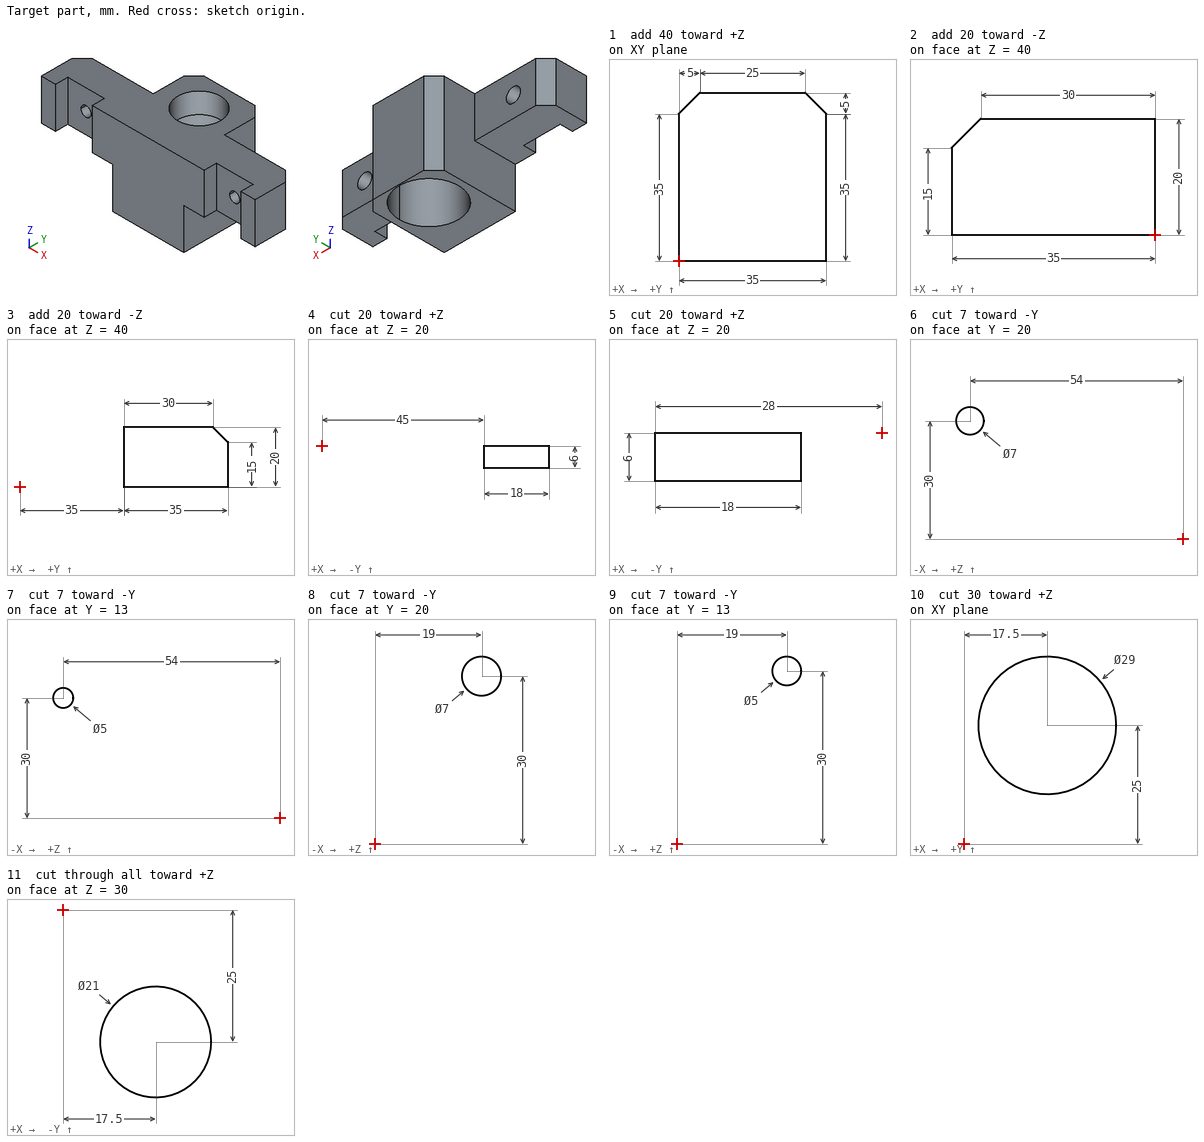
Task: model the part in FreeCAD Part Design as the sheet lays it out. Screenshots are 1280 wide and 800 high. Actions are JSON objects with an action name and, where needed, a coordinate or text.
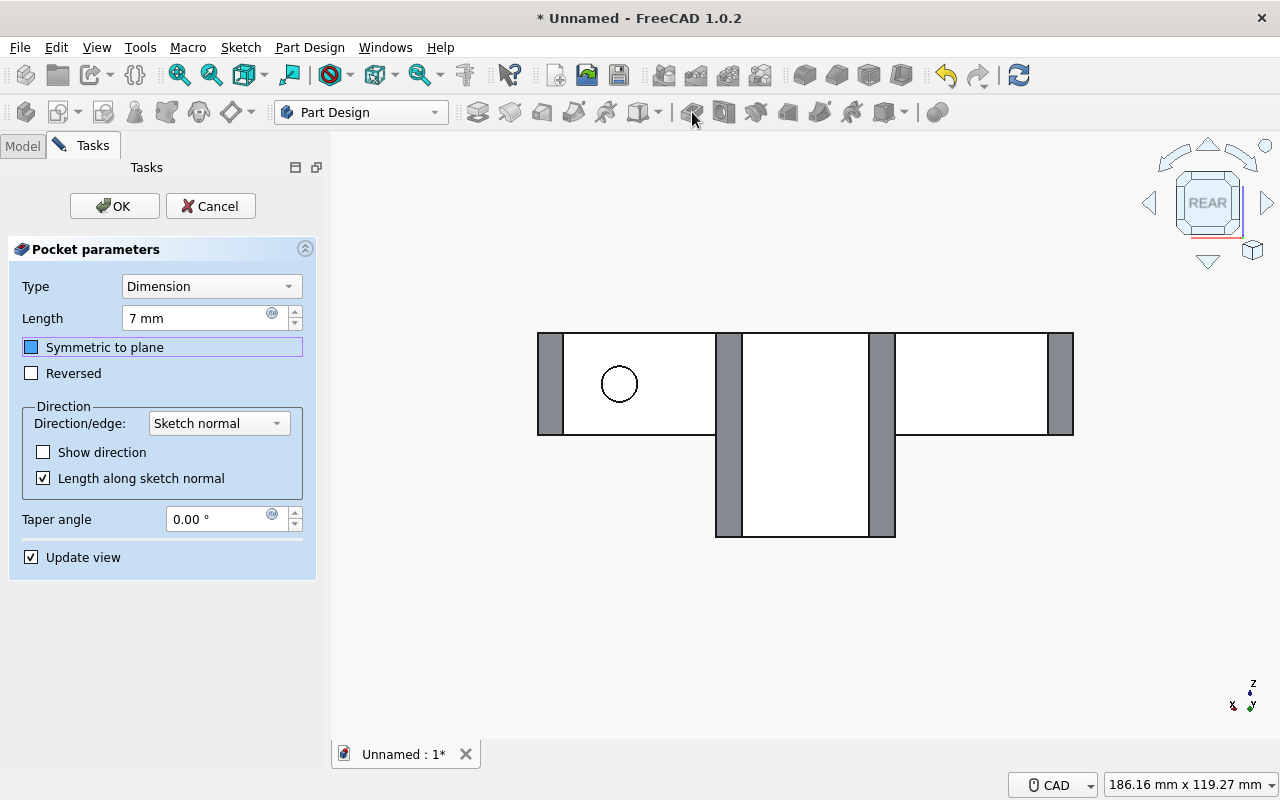
{"action": "left_click", "coordinate": [115, 206]}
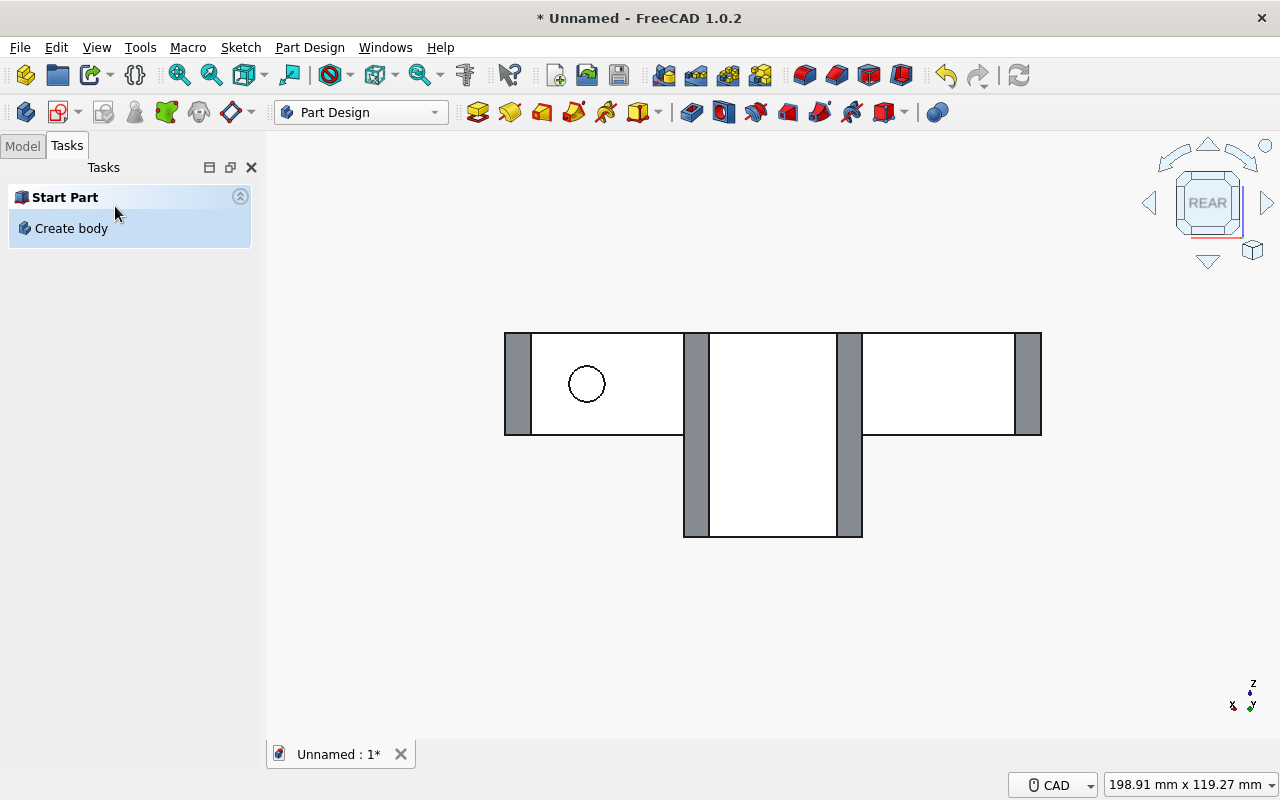
{"action": "left_click", "coordinate": [587, 383]}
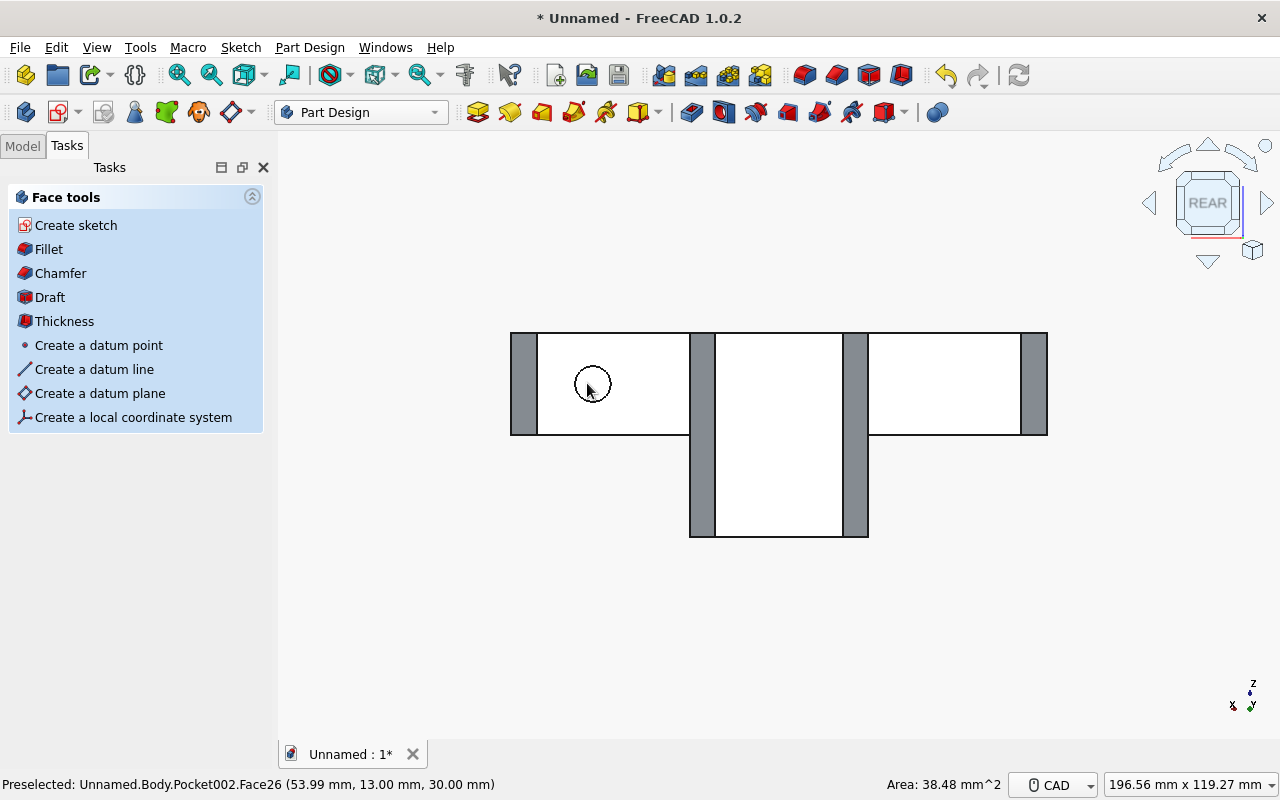
{"action": "left_click", "coordinate": [58, 112]}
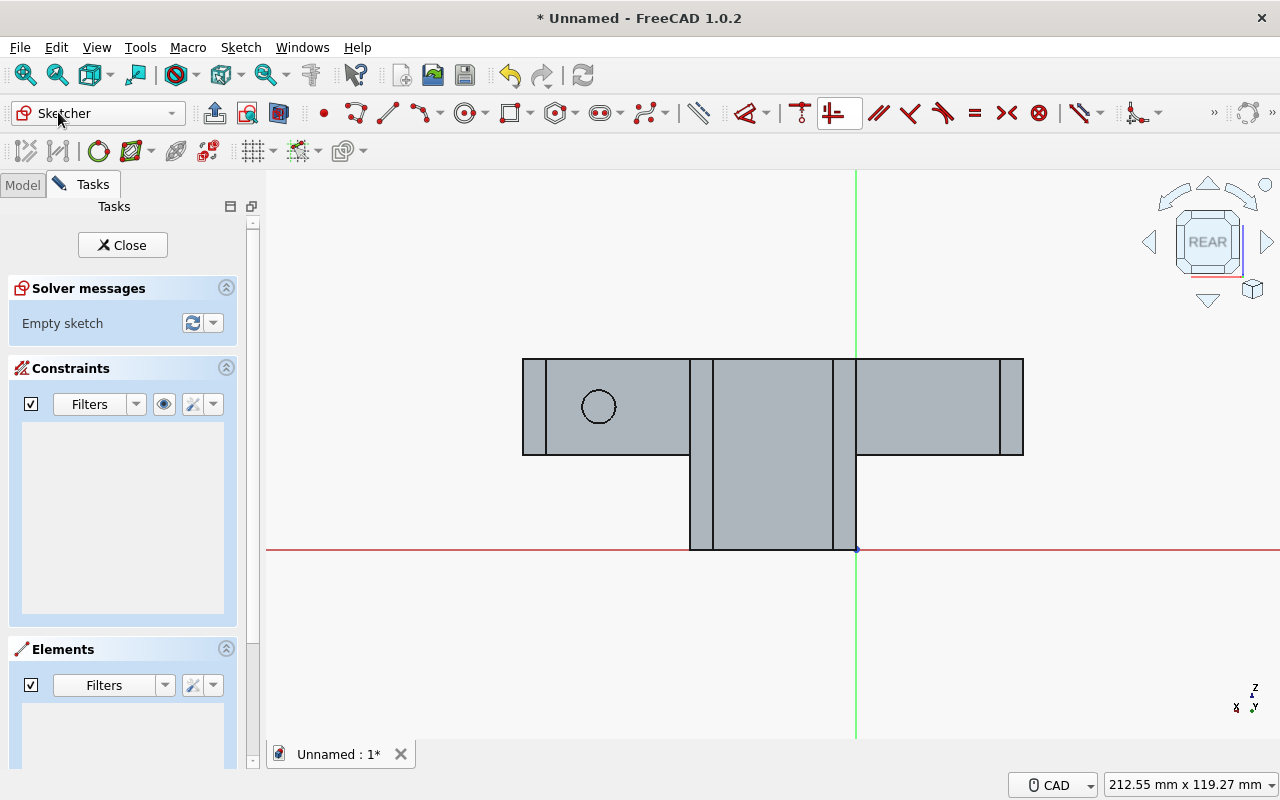
{"action": "scroll", "coordinate": [592, 404], "scroll_direction": "up", "scroll_amount": 14}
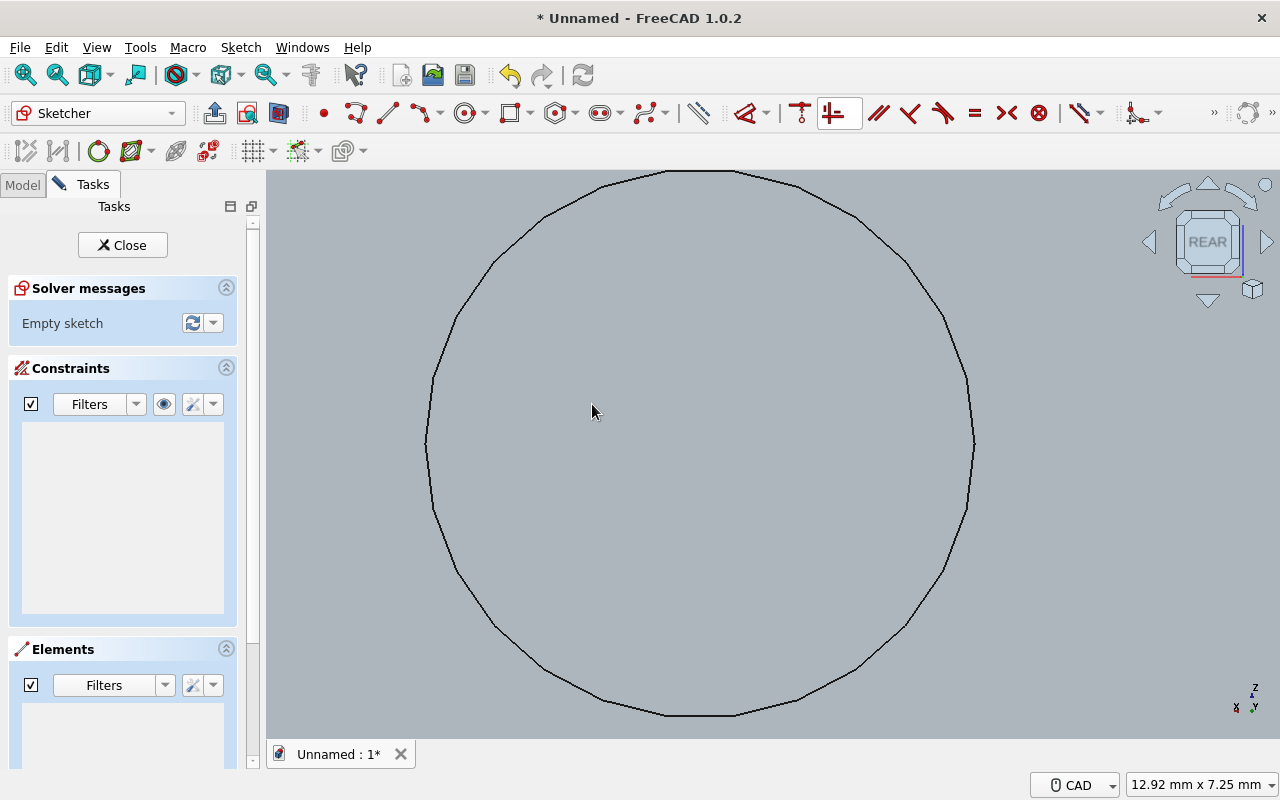
{"action": "left_click", "coordinate": [466, 114]}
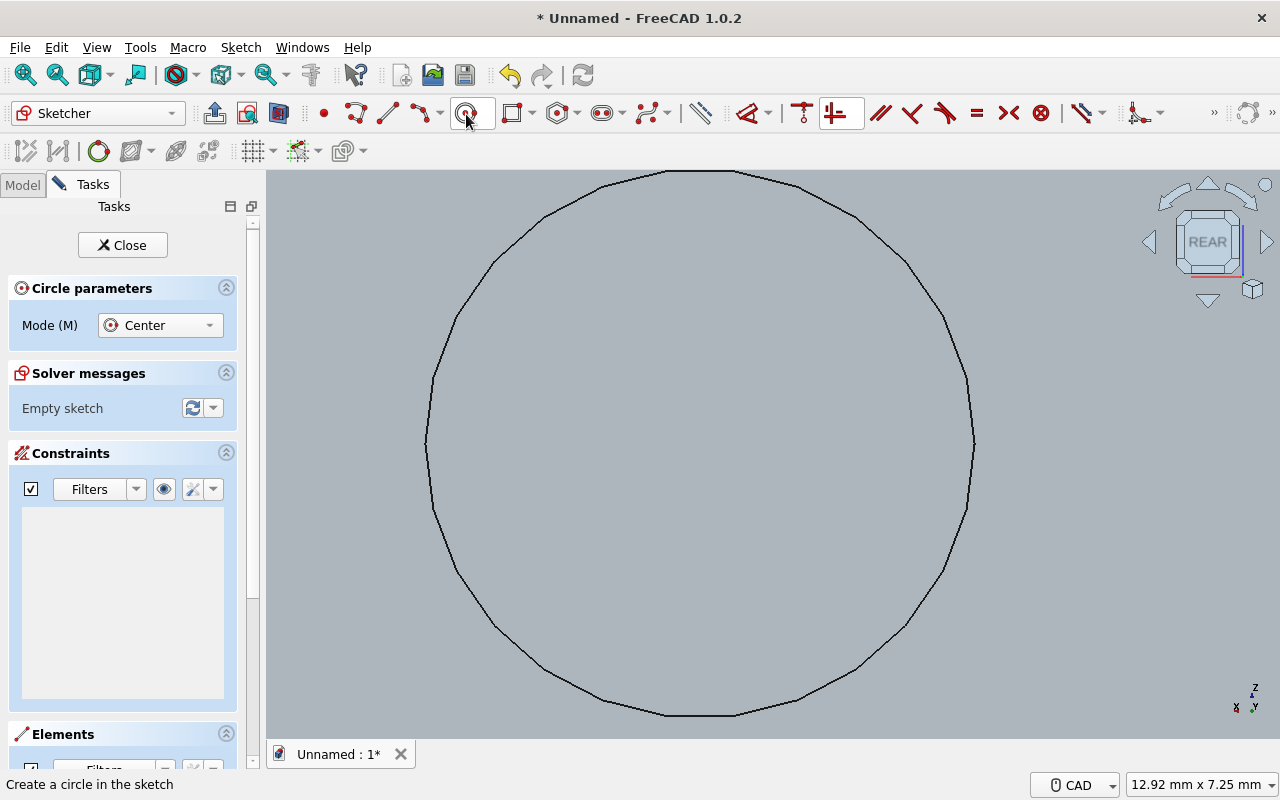
{"action": "left_click", "coordinate": [700, 444]}
{"action": "left_click", "coordinate": [839, 305]}
{"action": "key", "text": "Escape"}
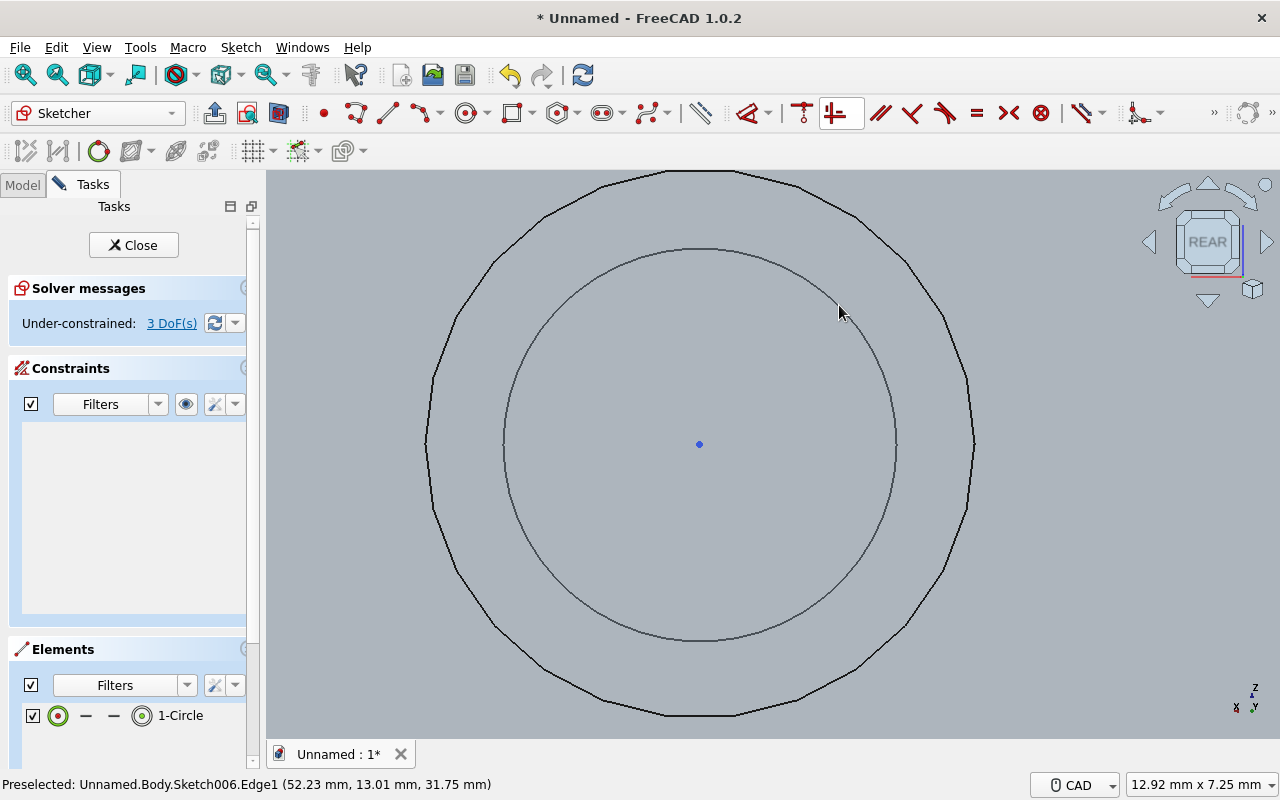
{"action": "left_click", "coordinate": [748, 114]}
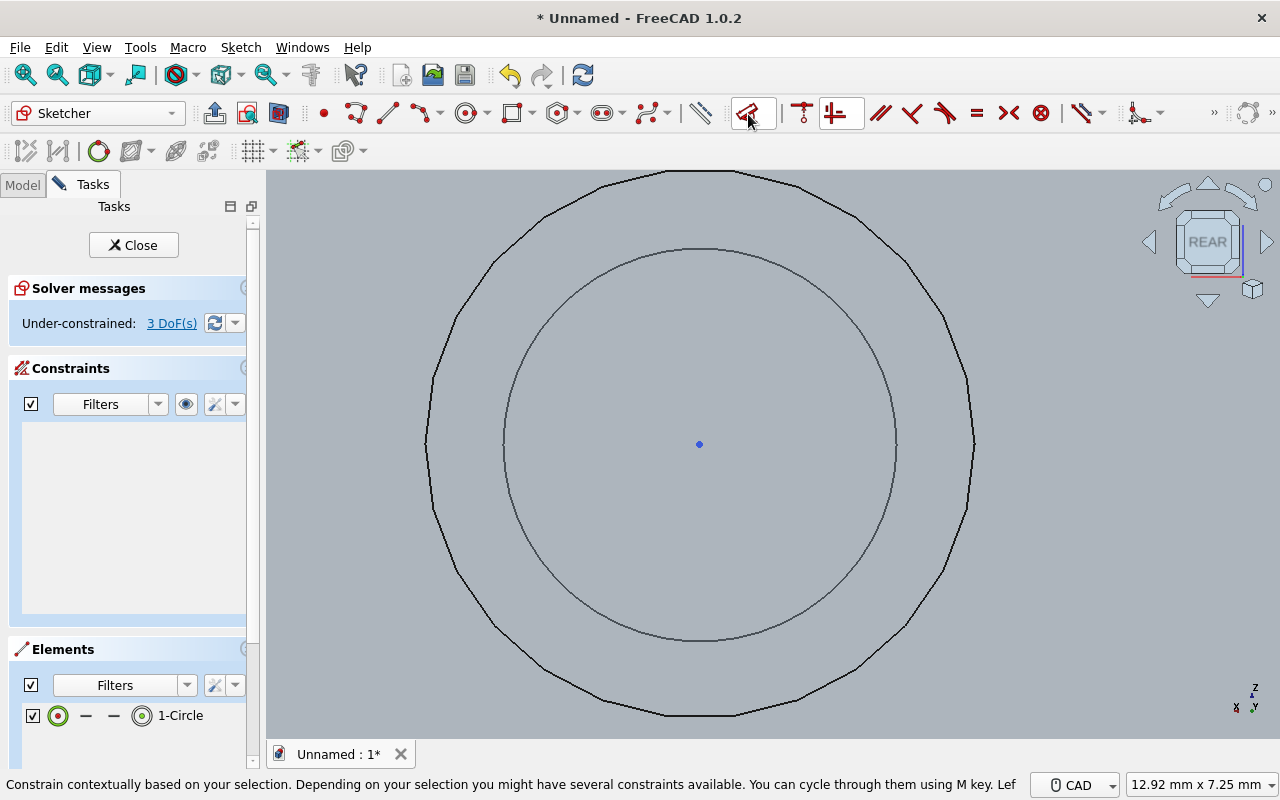
{"action": "left_click", "coordinate": [839, 306]}
{"action": "left_click", "coordinate": [862, 283]}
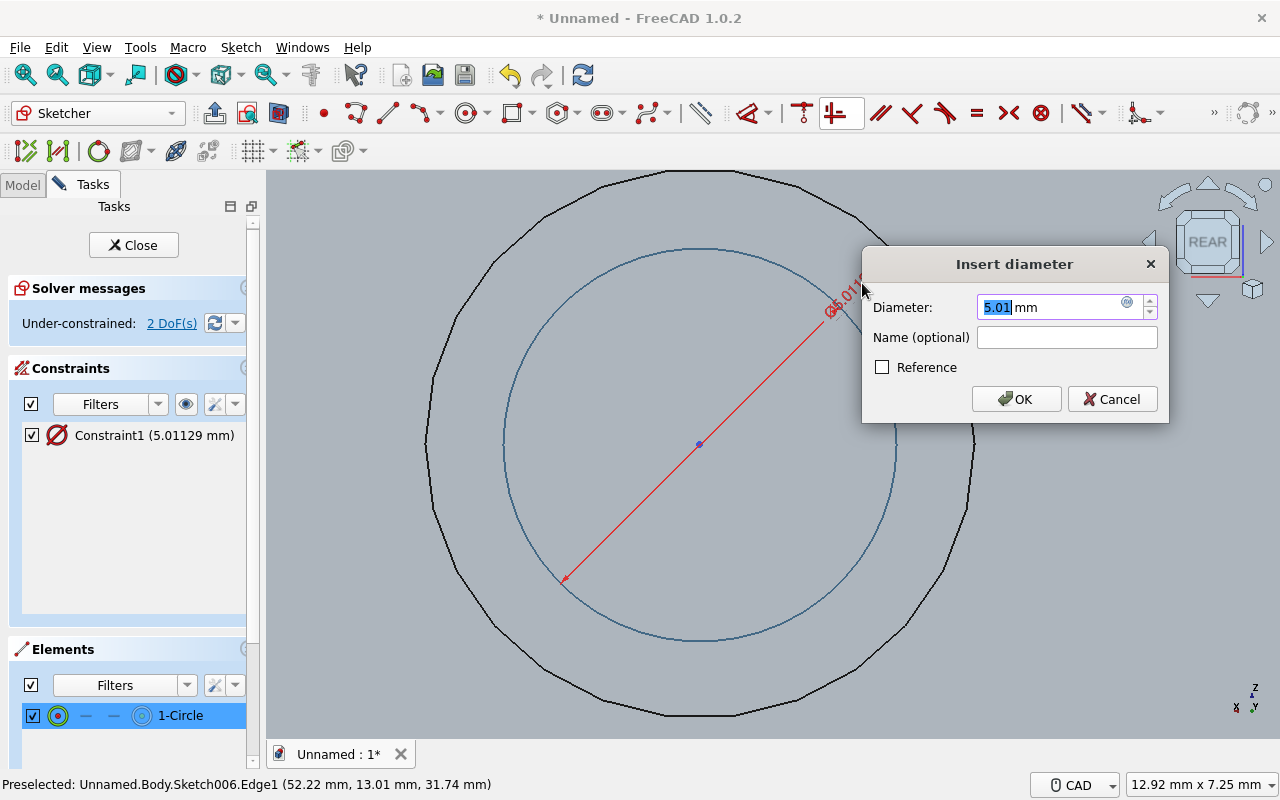
{"action": "type", "text": "5"}
{"action": "key", "text": "Return"}